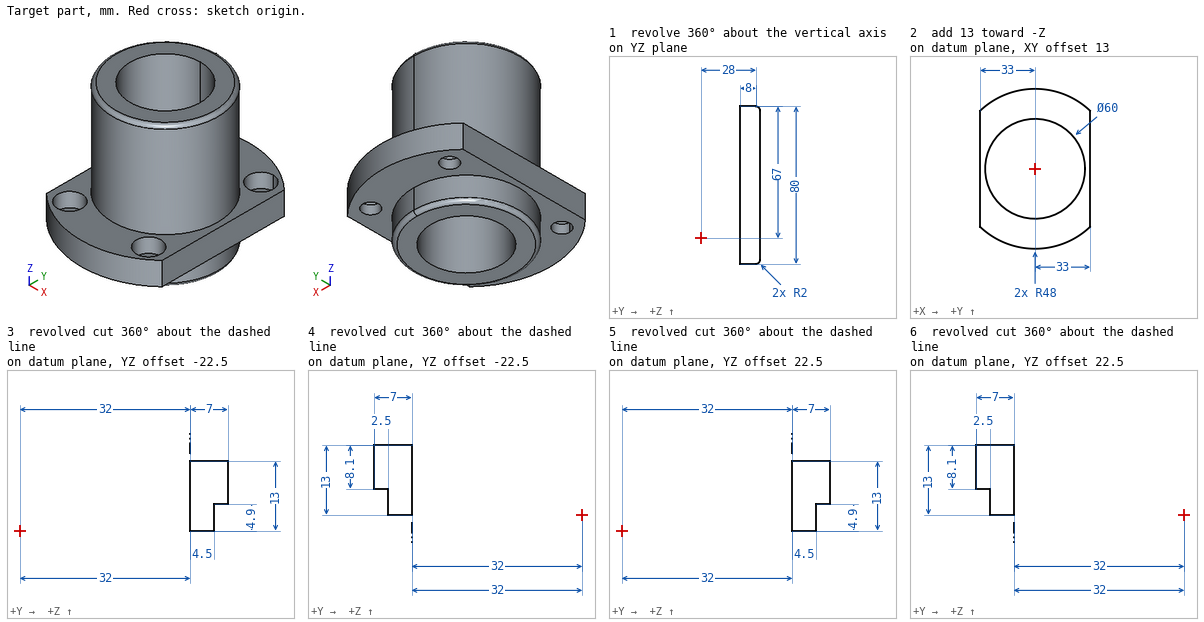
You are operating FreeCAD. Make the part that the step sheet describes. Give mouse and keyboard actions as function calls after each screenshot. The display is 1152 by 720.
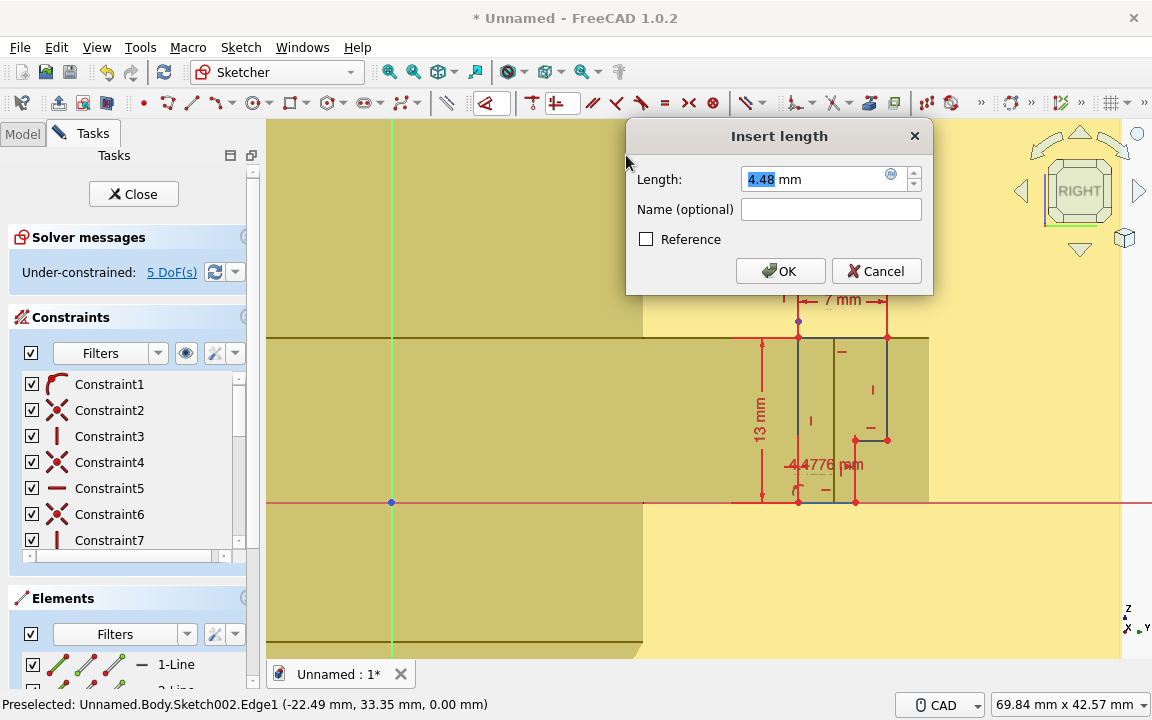
text(4.5)
key(Return)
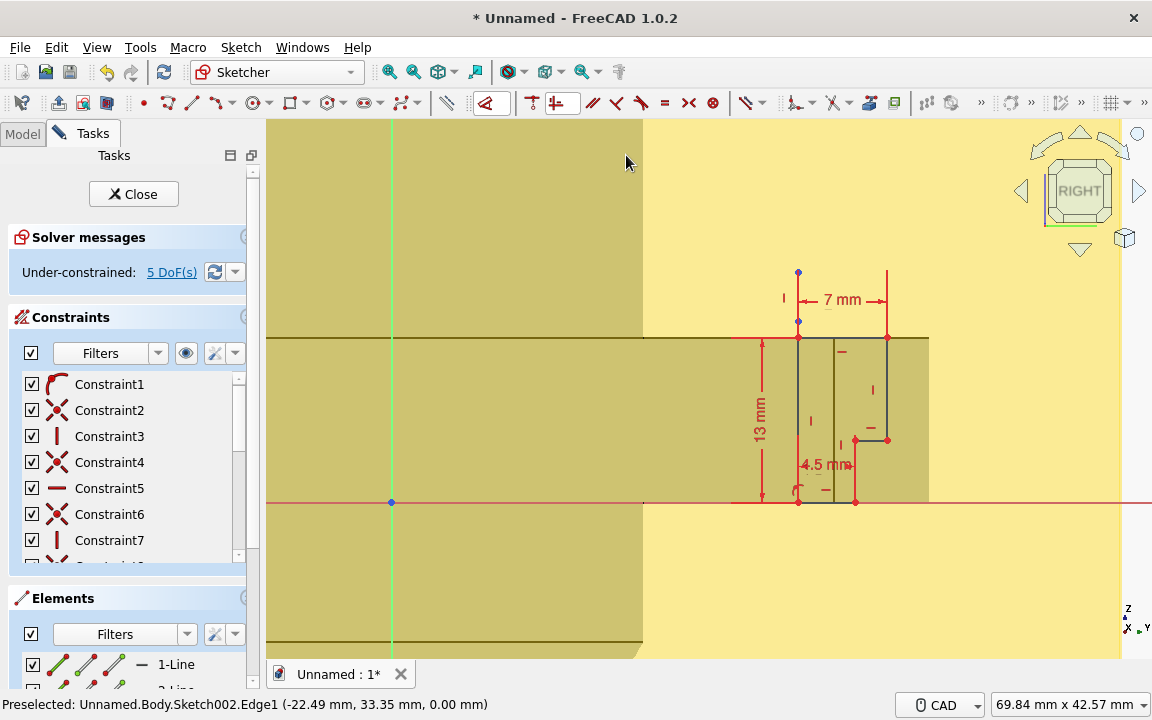
click(855, 484)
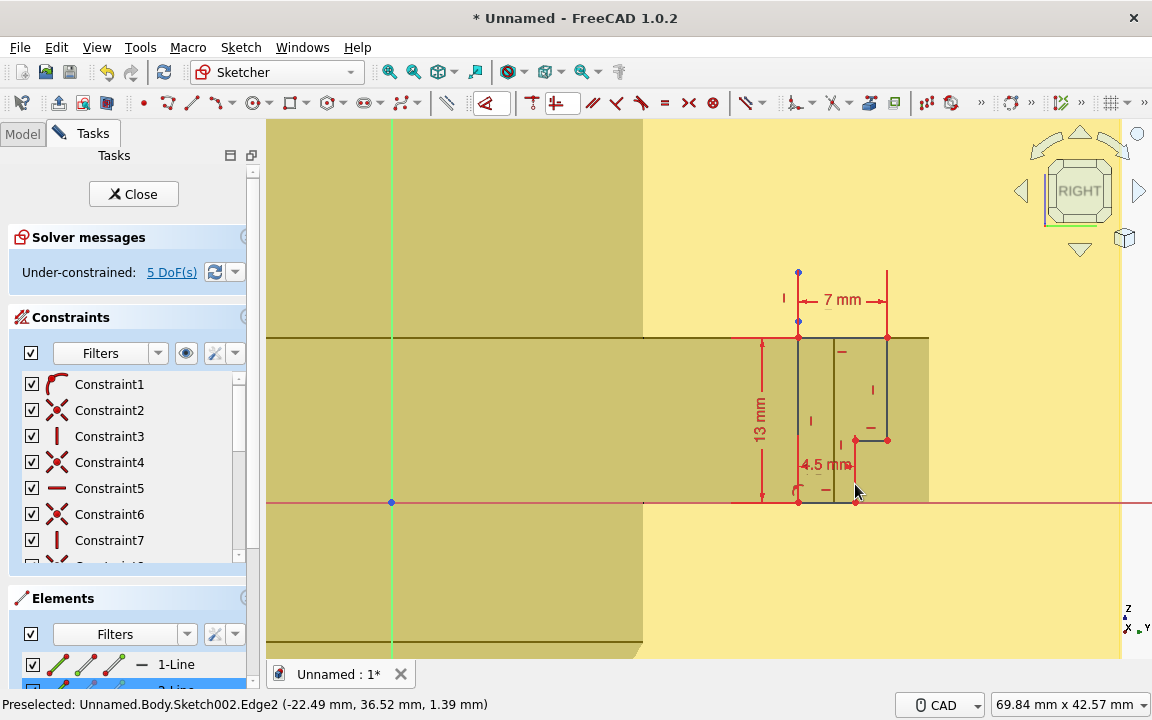
key(i)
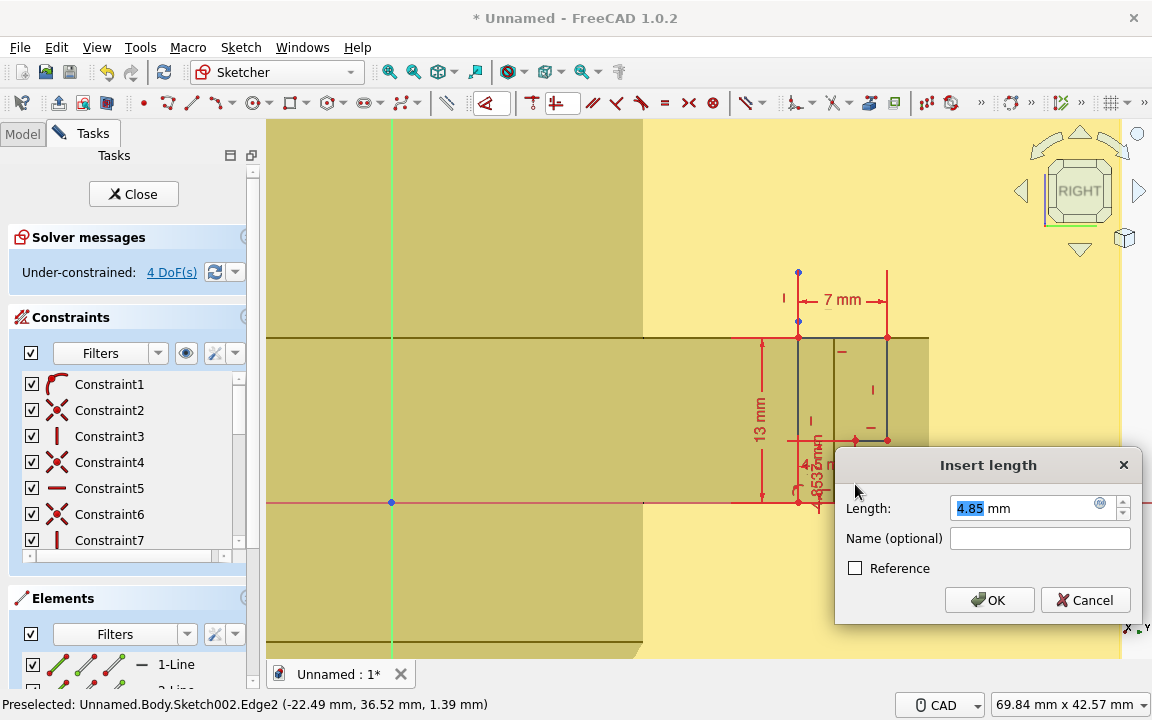
text(4.9)
key(Return)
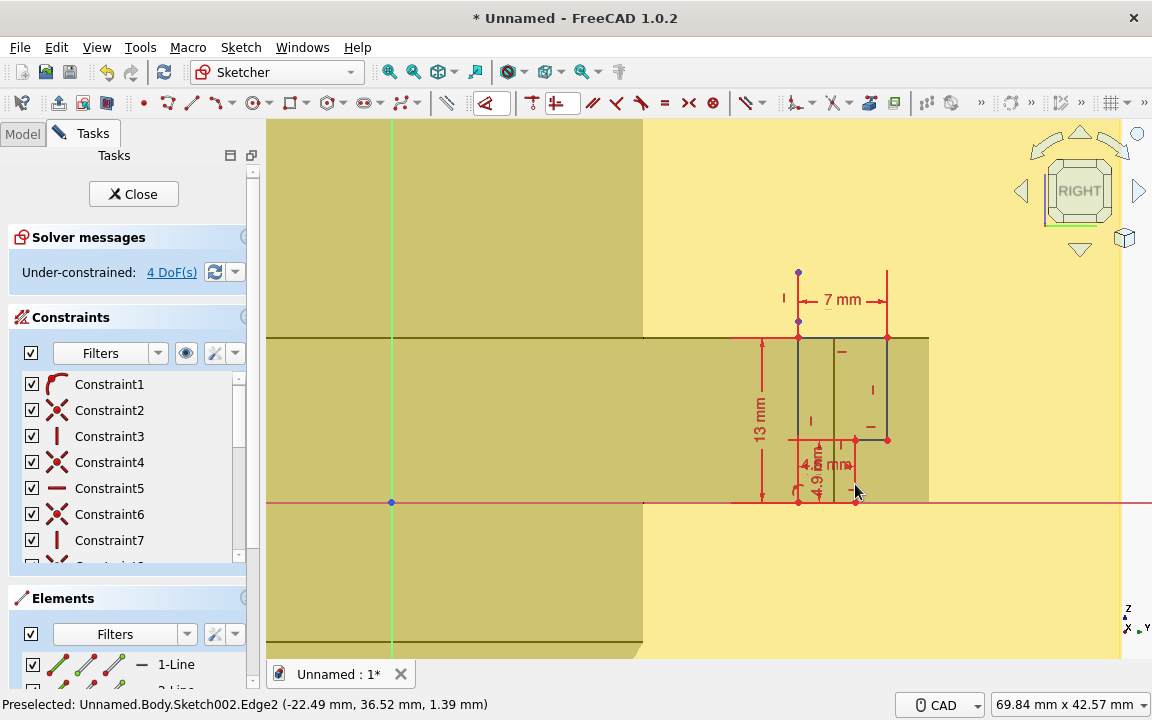
click(798, 503)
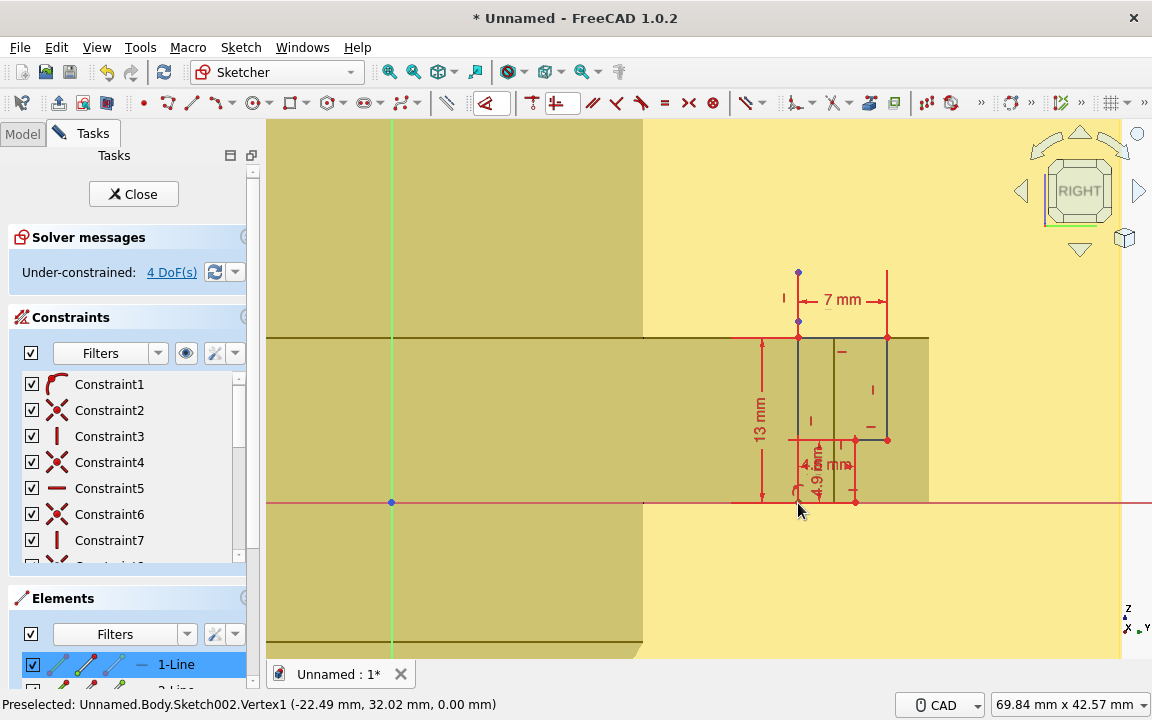
click(504, 104)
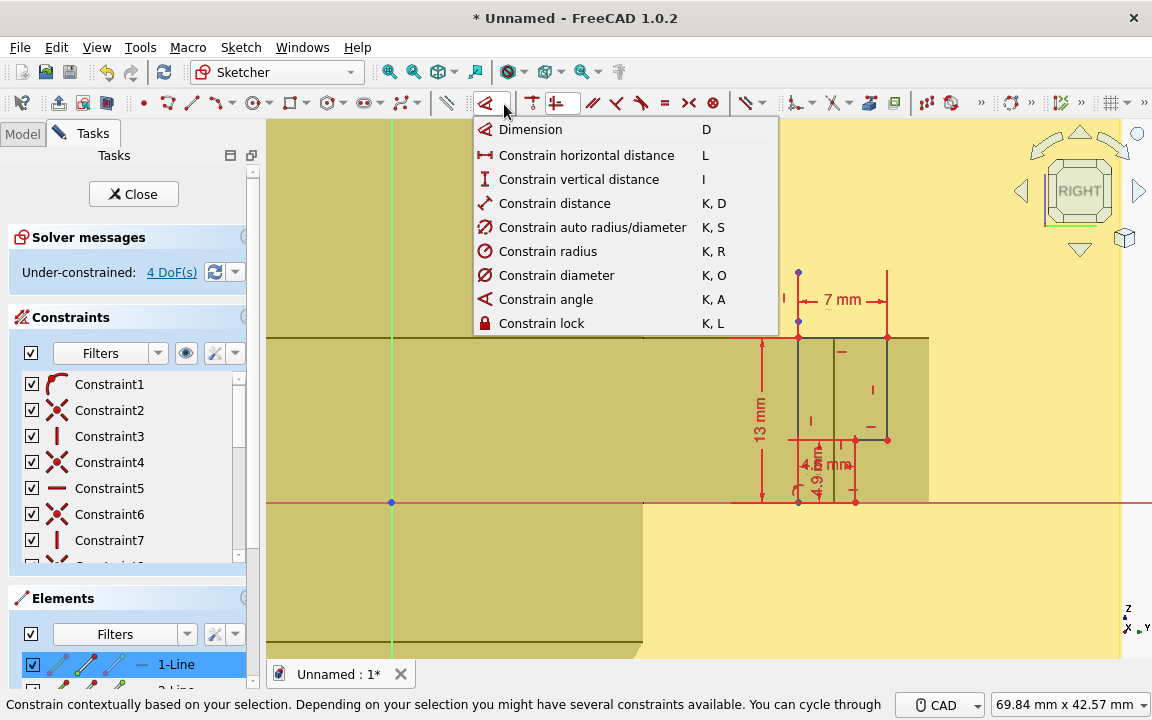
click(626, 155)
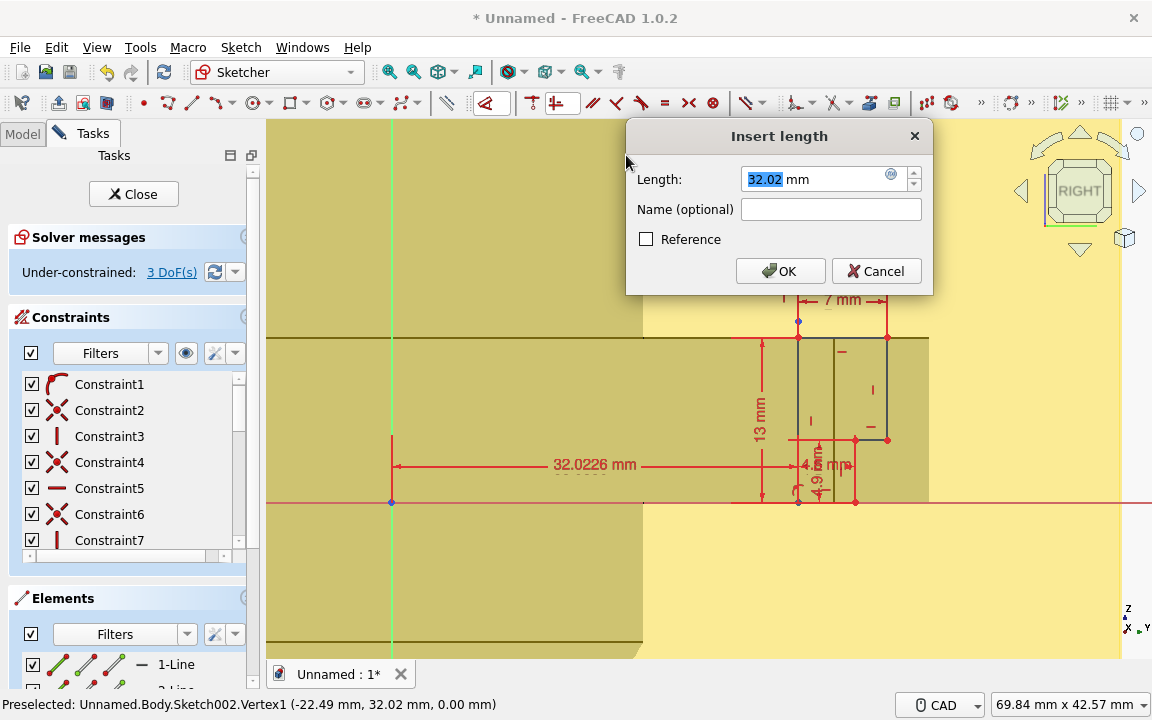
text(32)
key(Return)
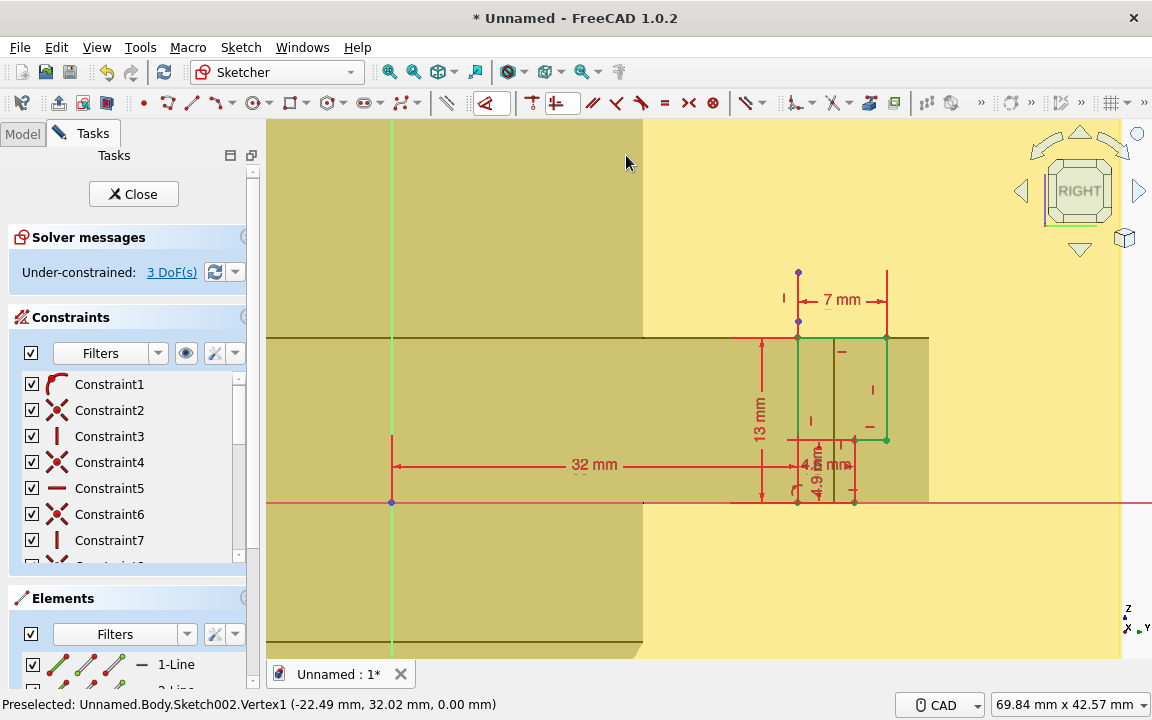
click(798, 322)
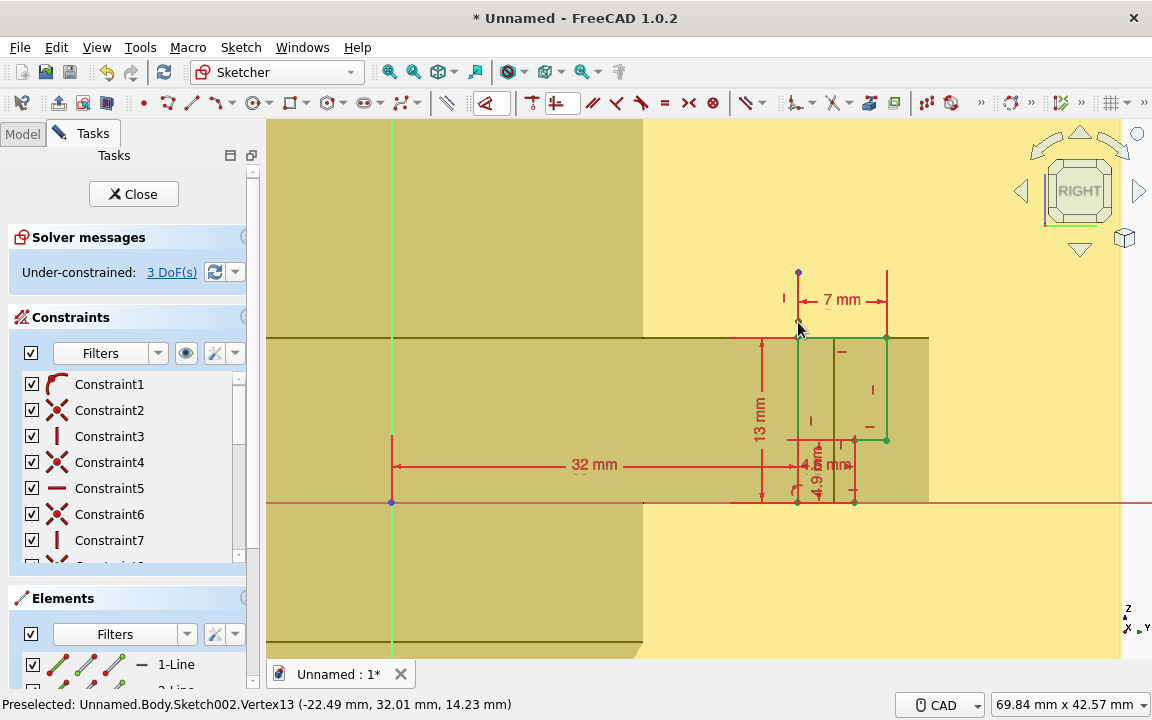
click(504, 104)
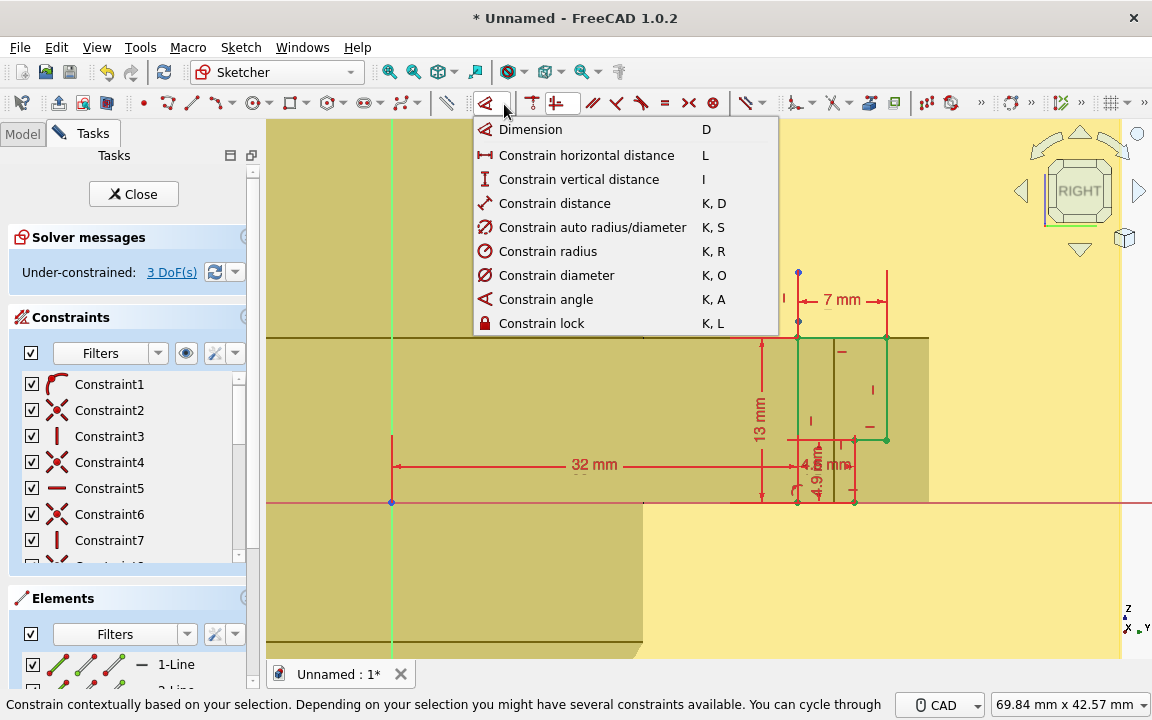
click(626, 155)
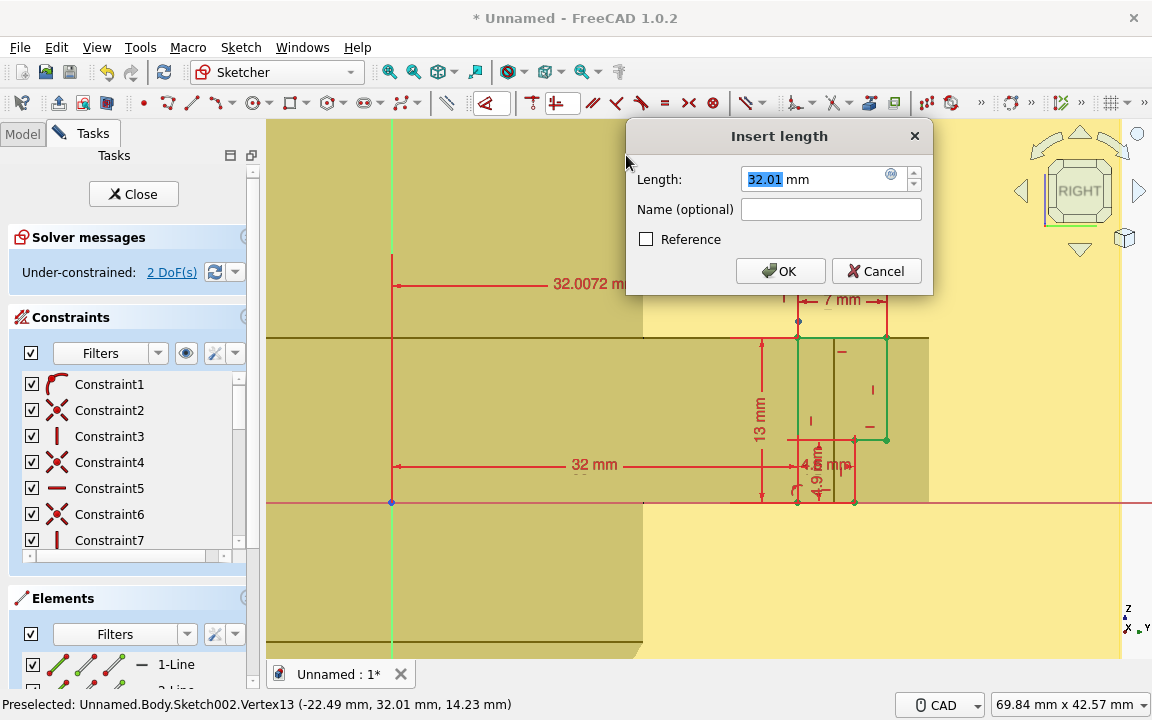
text(32)
key(Return)